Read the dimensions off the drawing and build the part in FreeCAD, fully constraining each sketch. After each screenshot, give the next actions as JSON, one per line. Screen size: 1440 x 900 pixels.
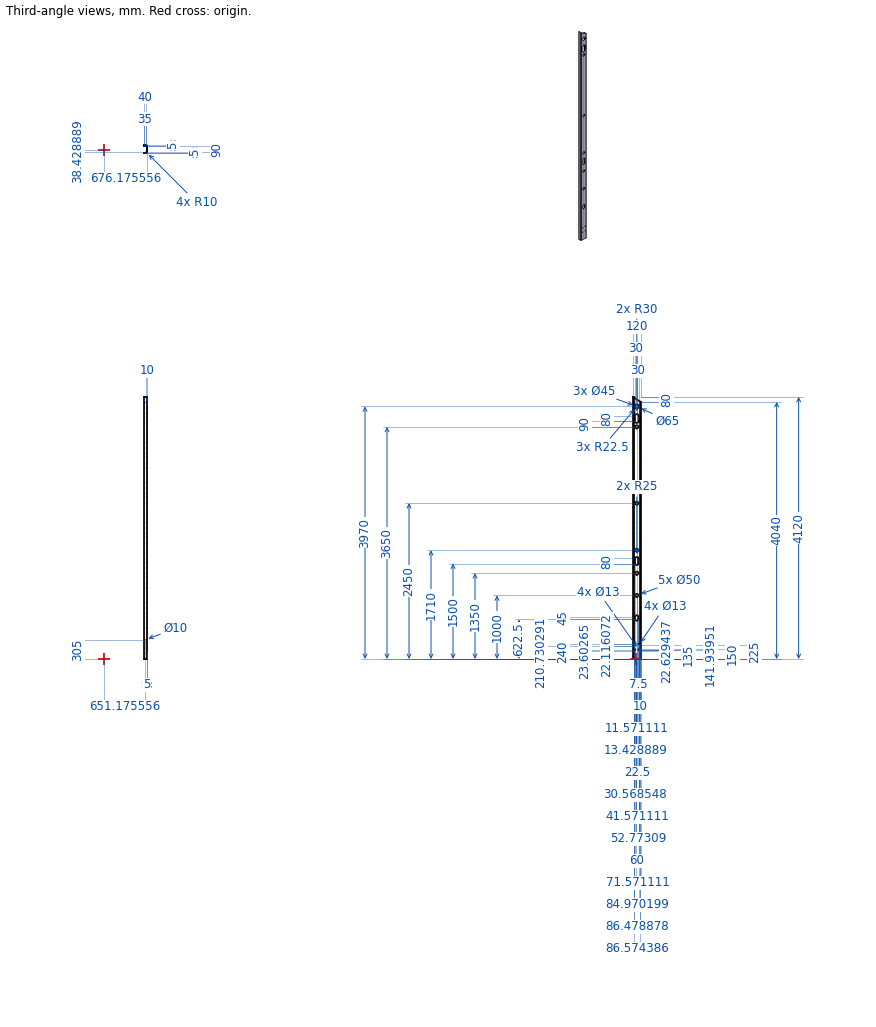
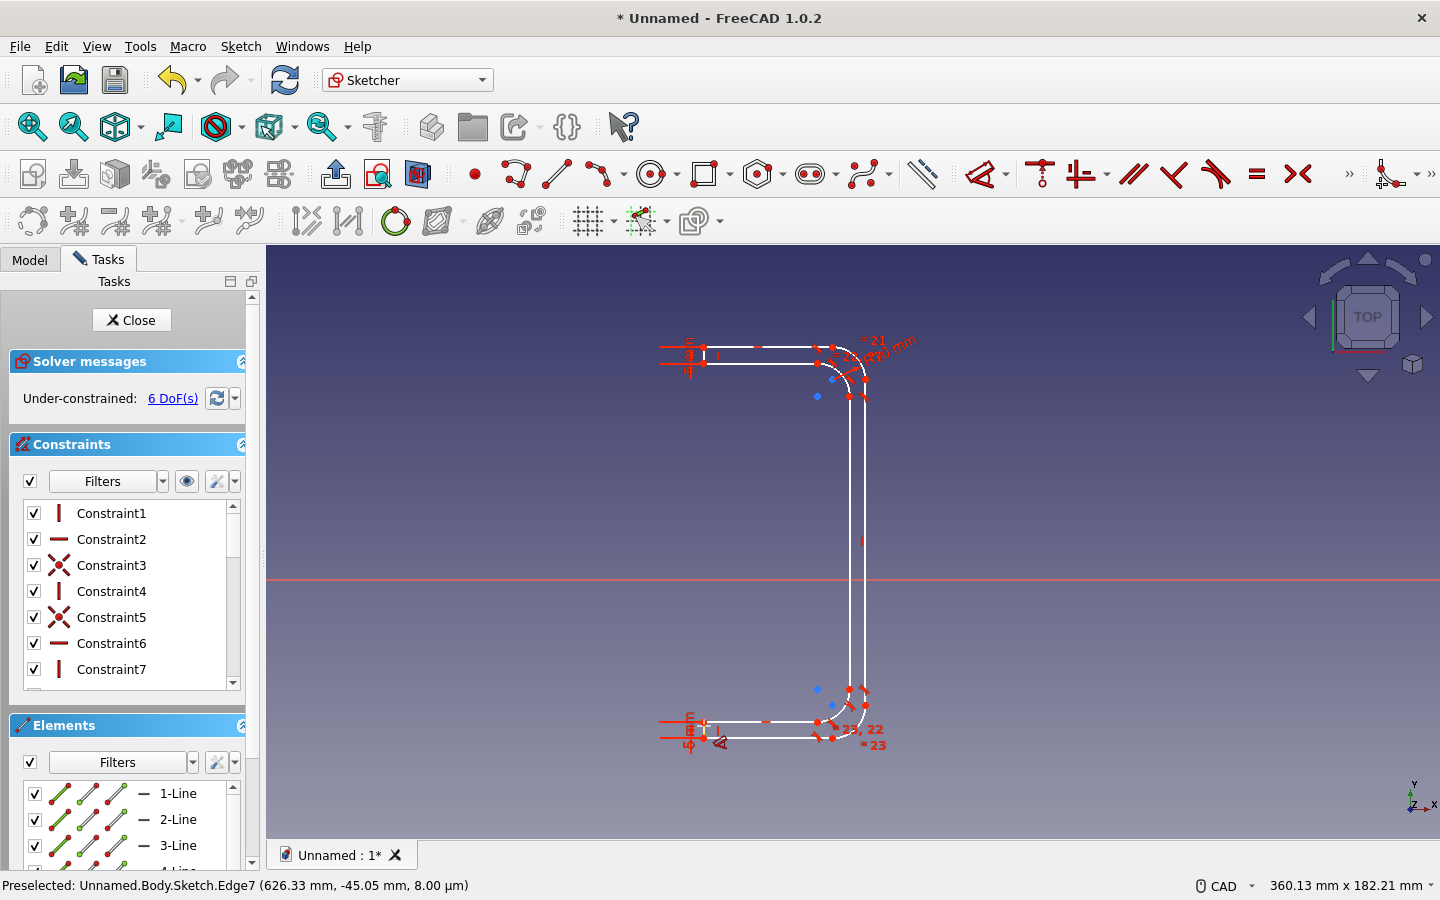
{"action": "left_click", "coordinate": [794, 347]}
{"action": "left_click", "coordinate": [768, 313]}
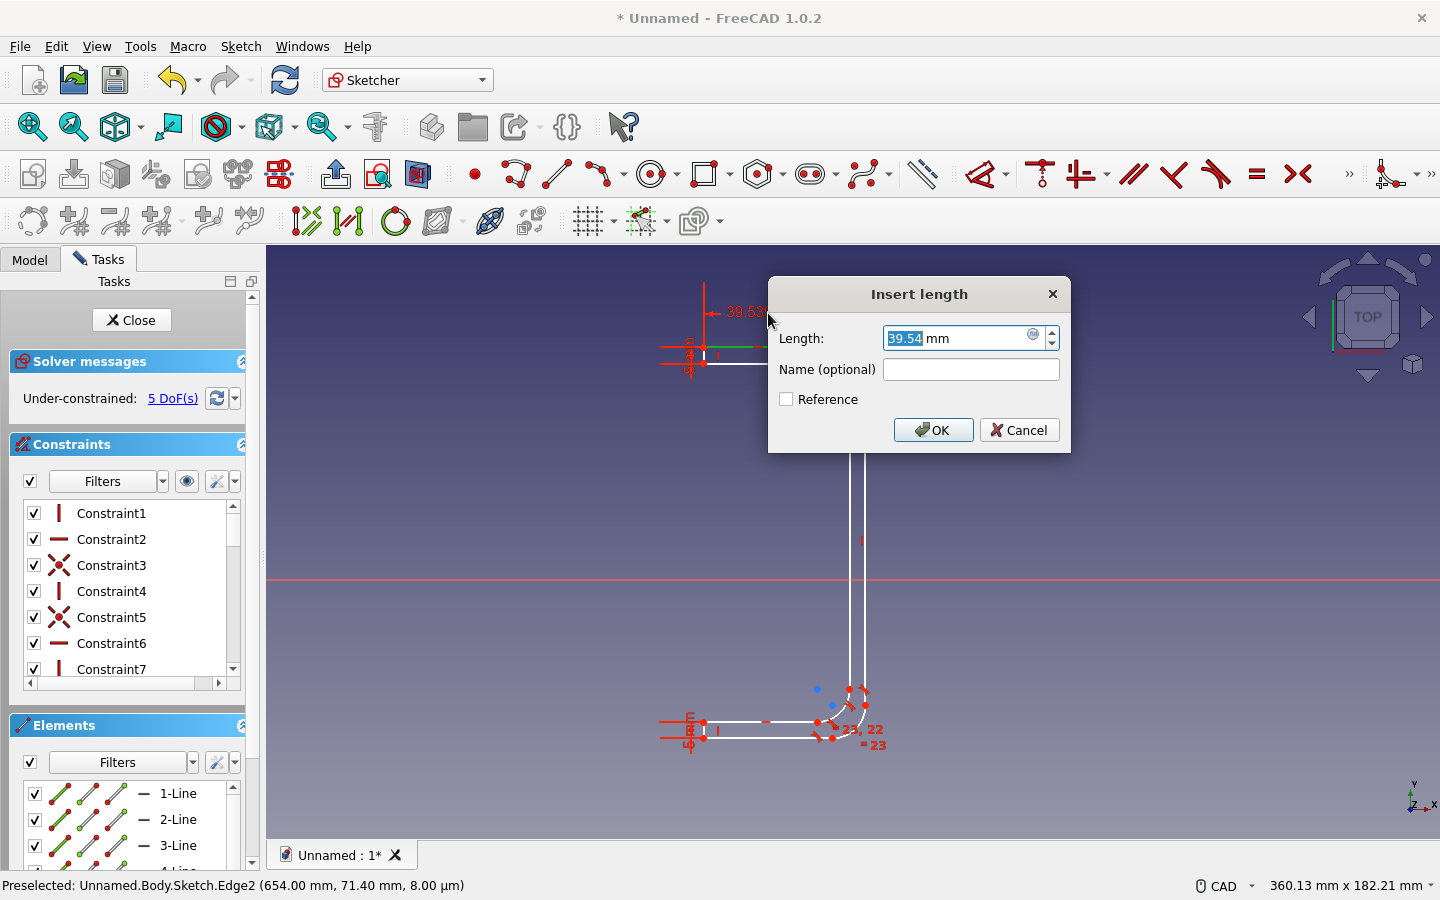
{"action": "type", "text": "40"}
{"action": "key", "text": "Return"}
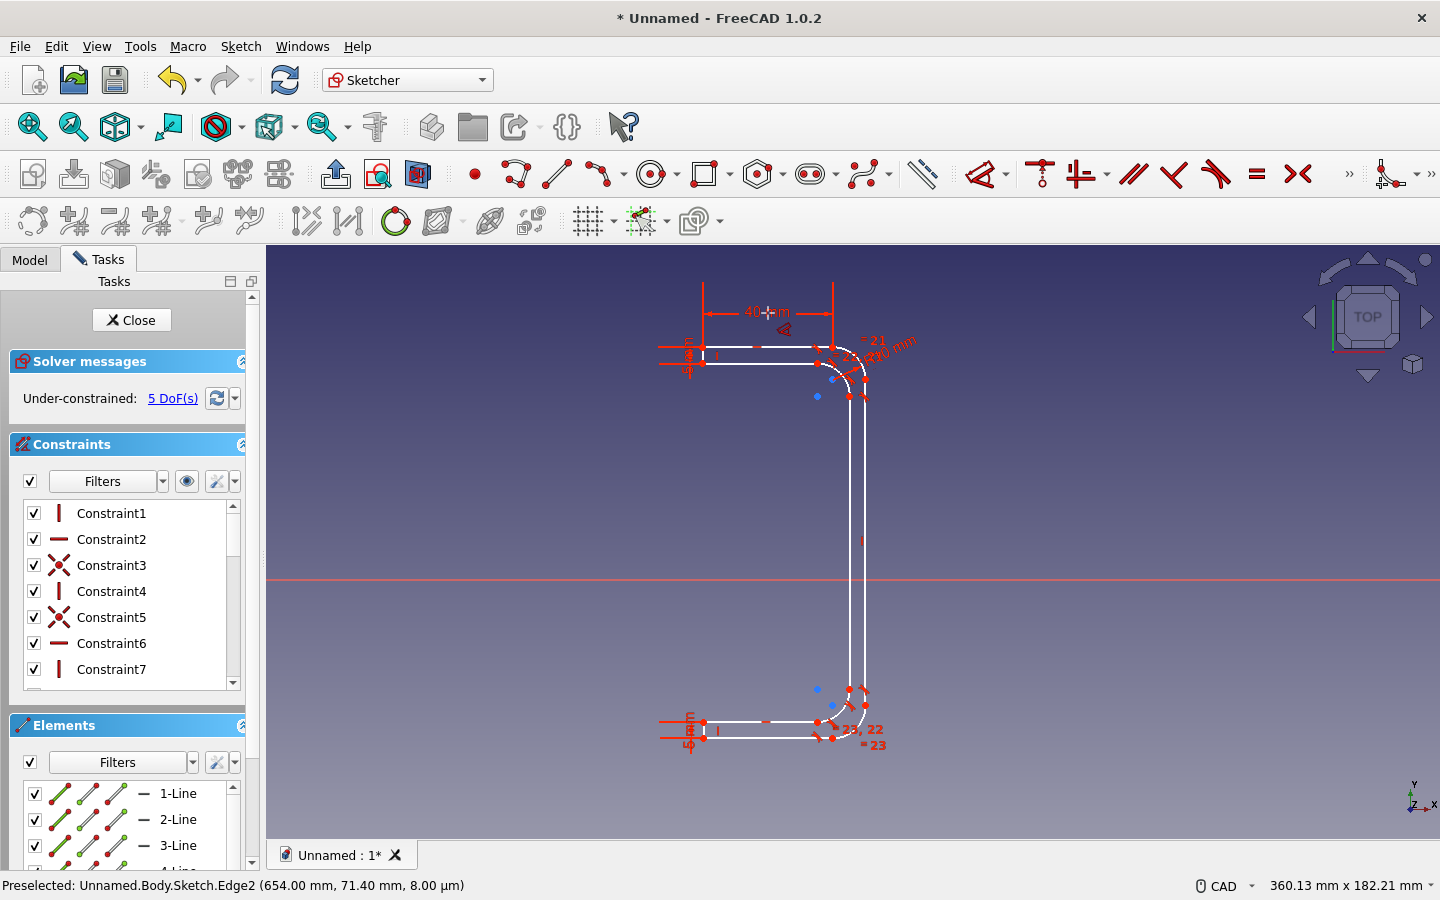
{"action": "left_click", "coordinate": [737, 364]}
{"action": "left_click", "coordinate": [760, 398]}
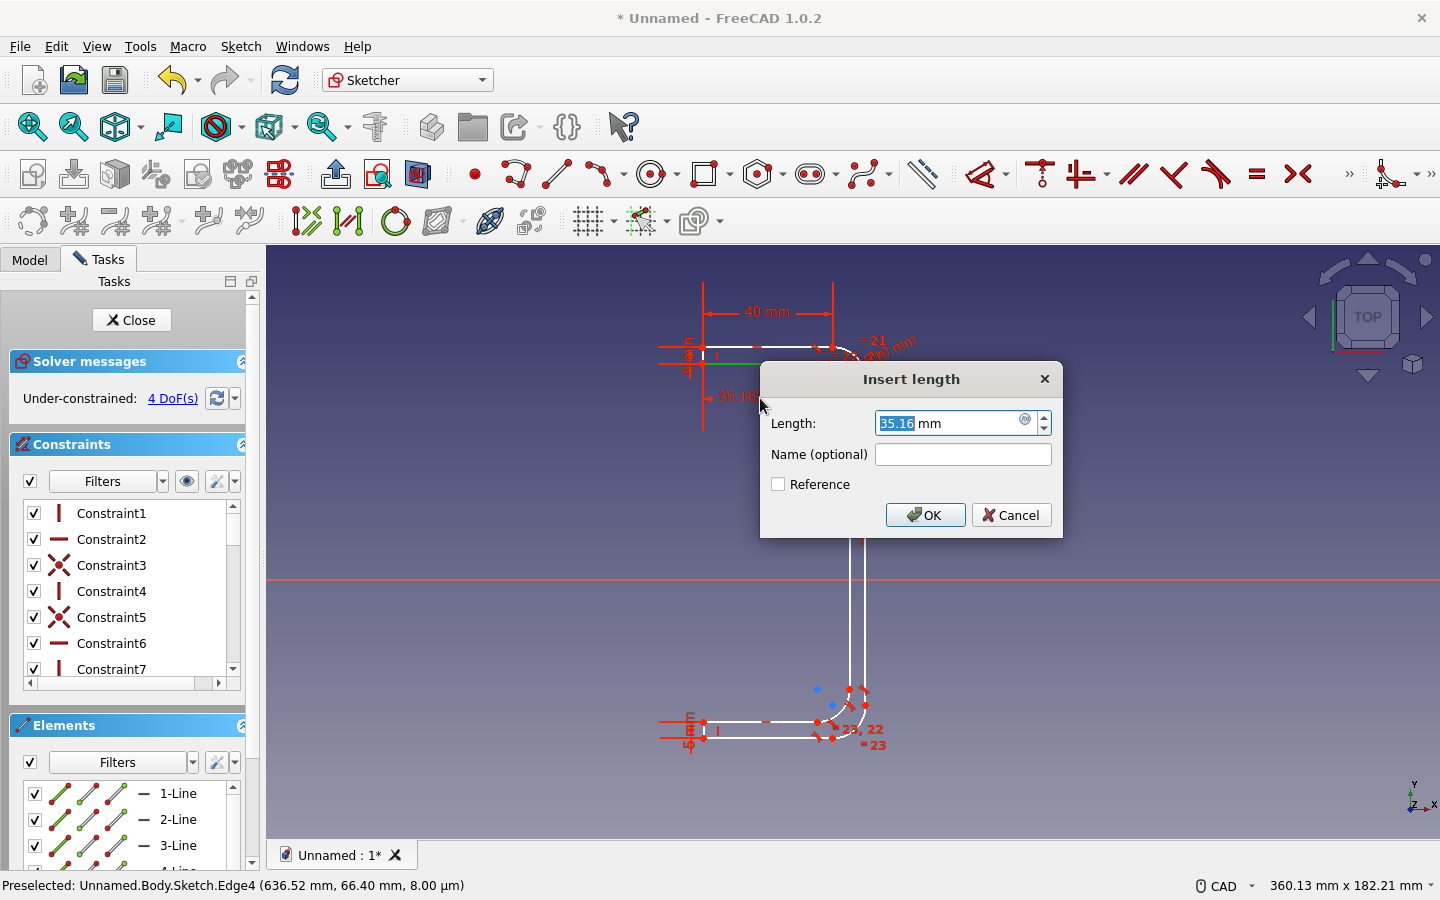
{"action": "type", "text": "35"}
{"action": "key", "text": "Return"}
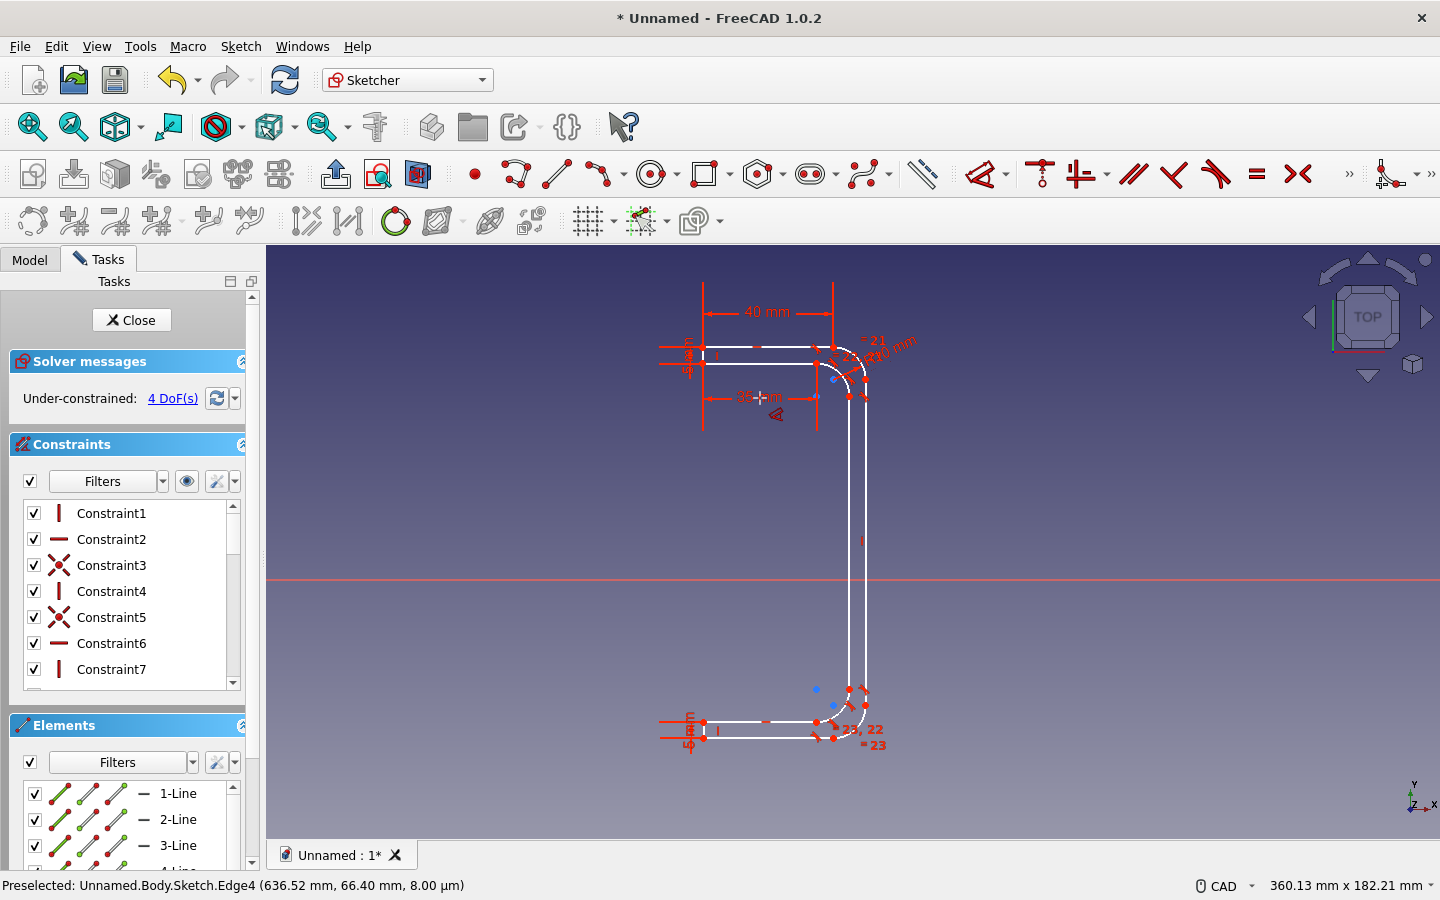
{"action": "left_click", "coordinate": [849, 484]}
{"action": "left_click", "coordinate": [883, 543]}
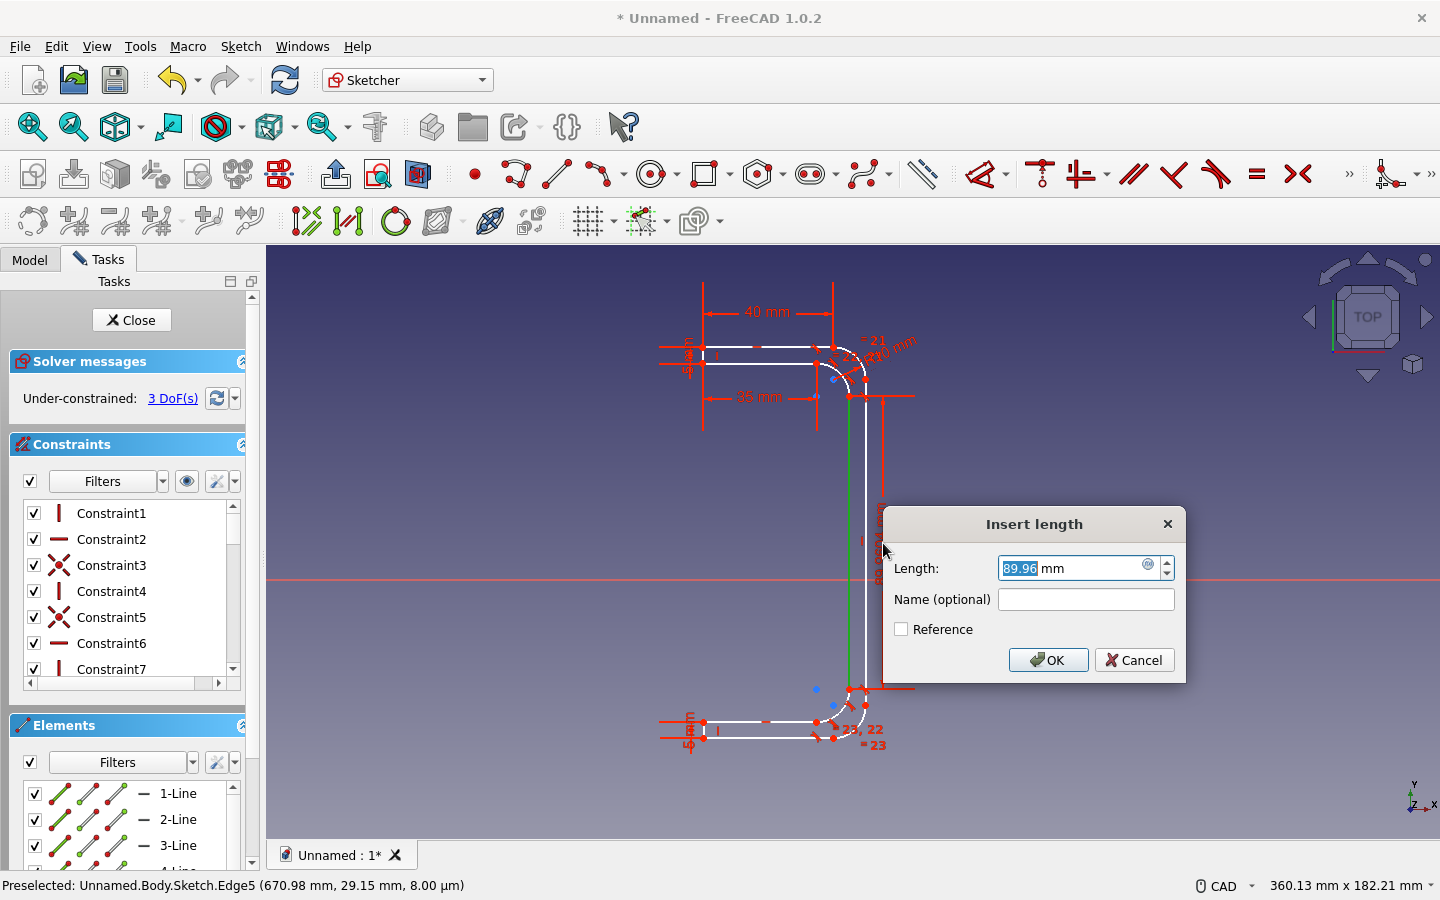
{"action": "type", "text": "90"}
{"action": "key", "text": "Return"}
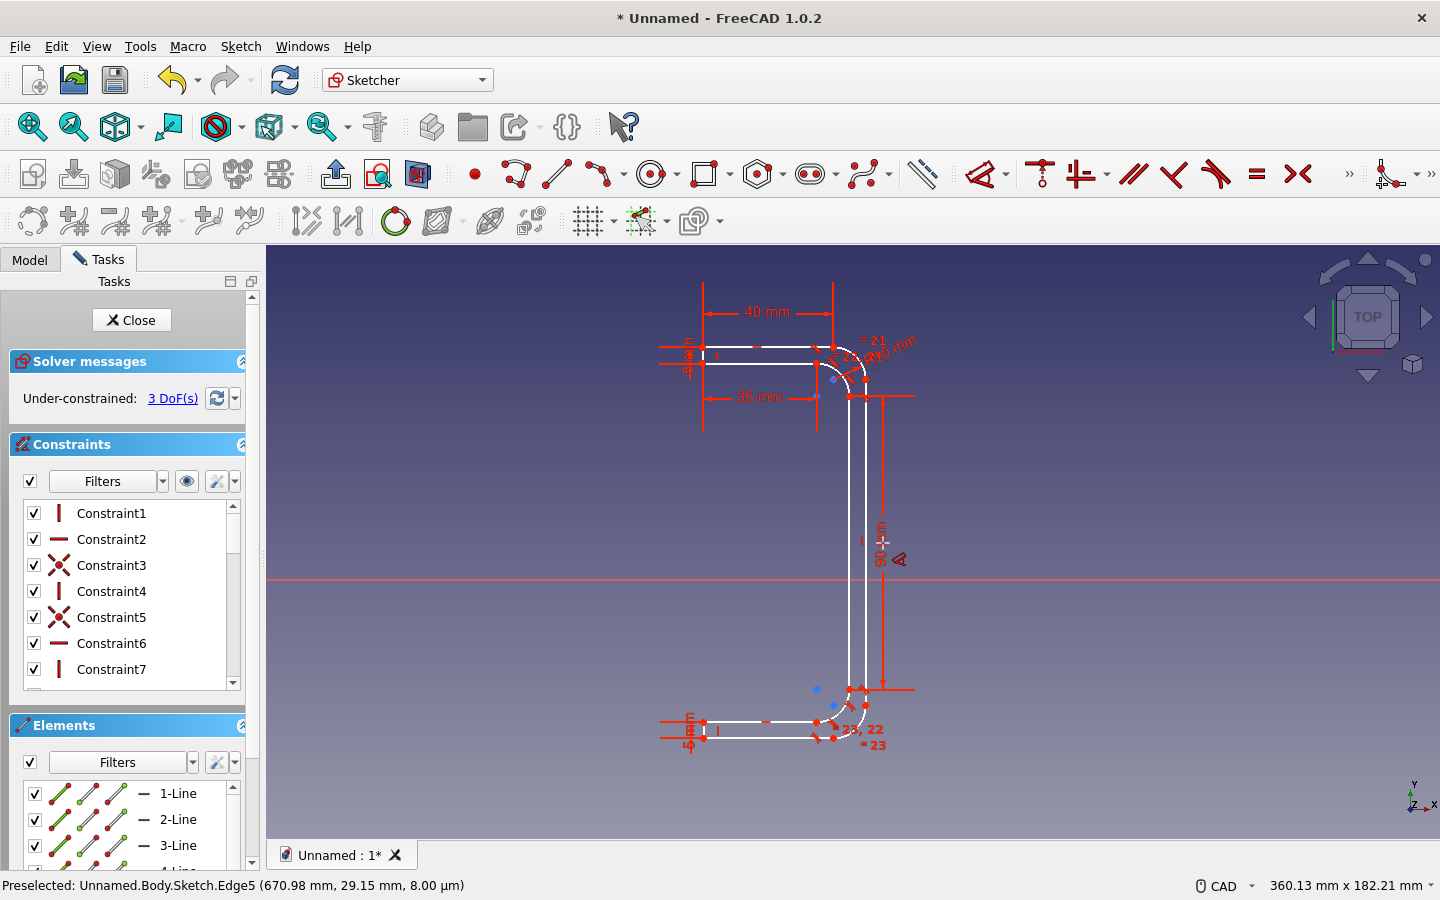
{"action": "left_click", "coordinate": [783, 722]}
{"action": "left_click", "coordinate": [760, 756]}